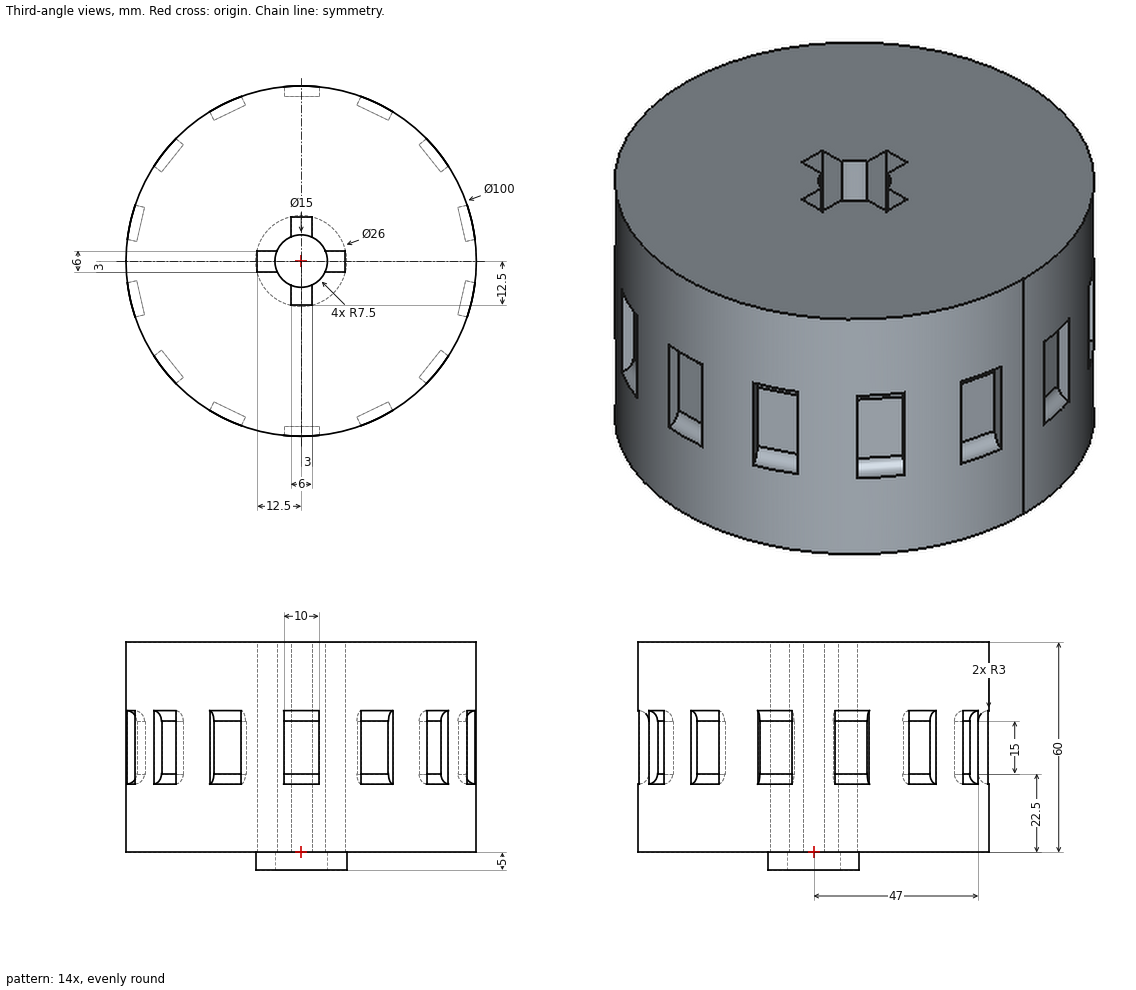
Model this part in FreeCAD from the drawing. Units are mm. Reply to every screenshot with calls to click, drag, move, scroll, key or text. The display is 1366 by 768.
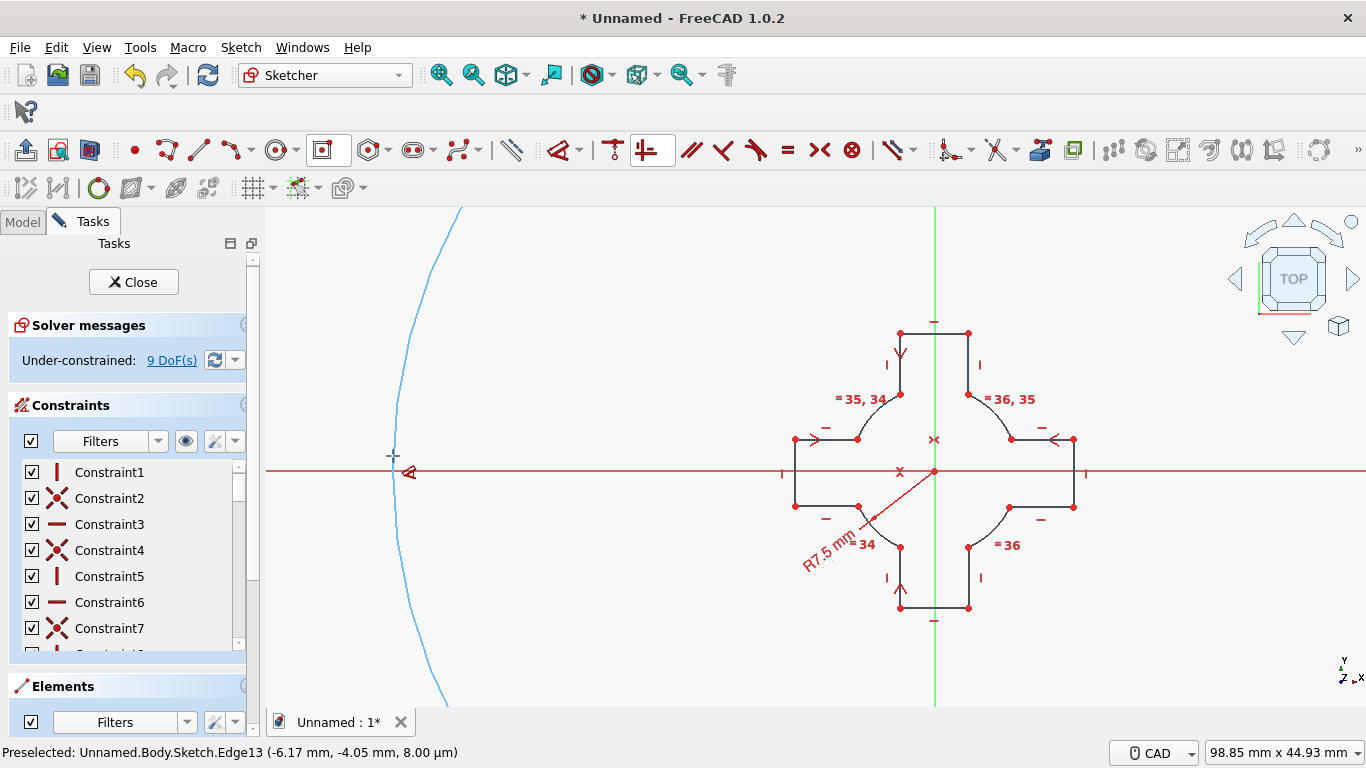
click(393, 456)
click(361, 455)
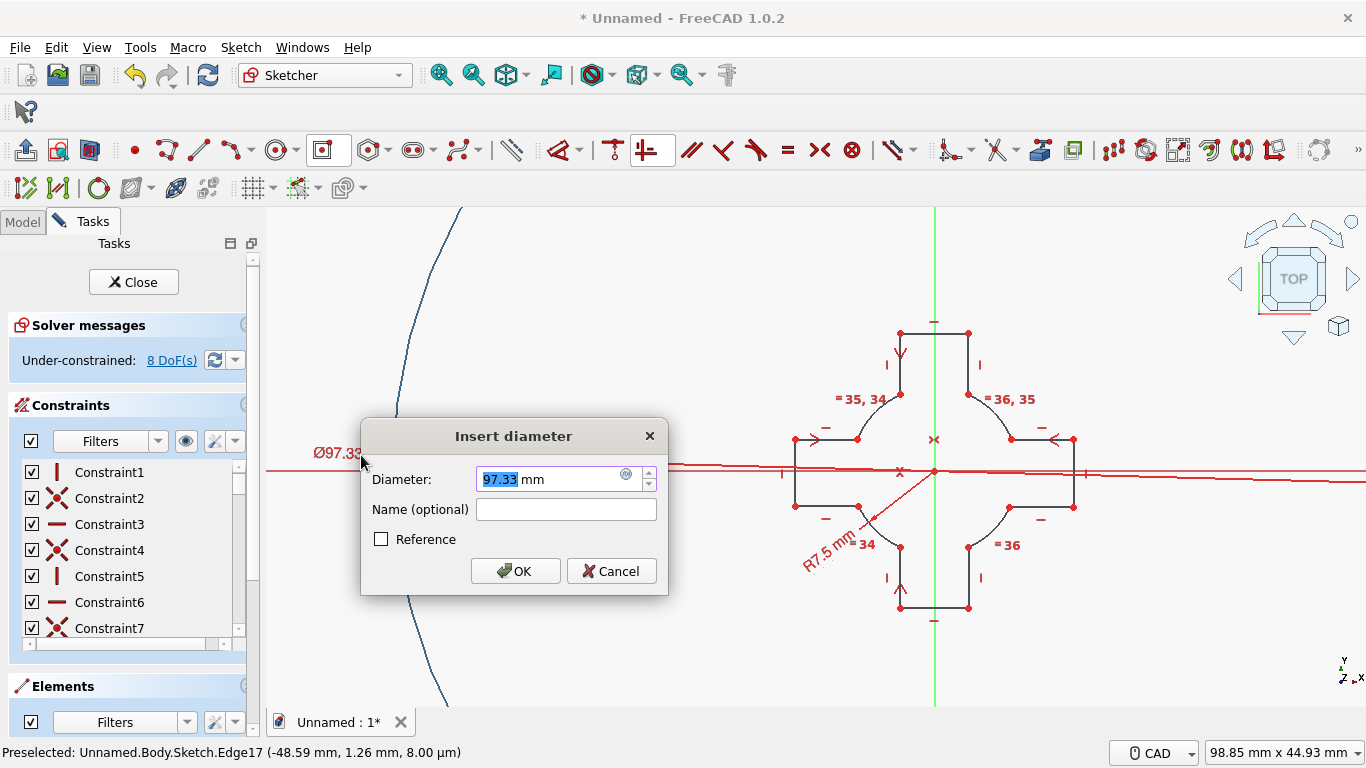
text(100)
key(Return)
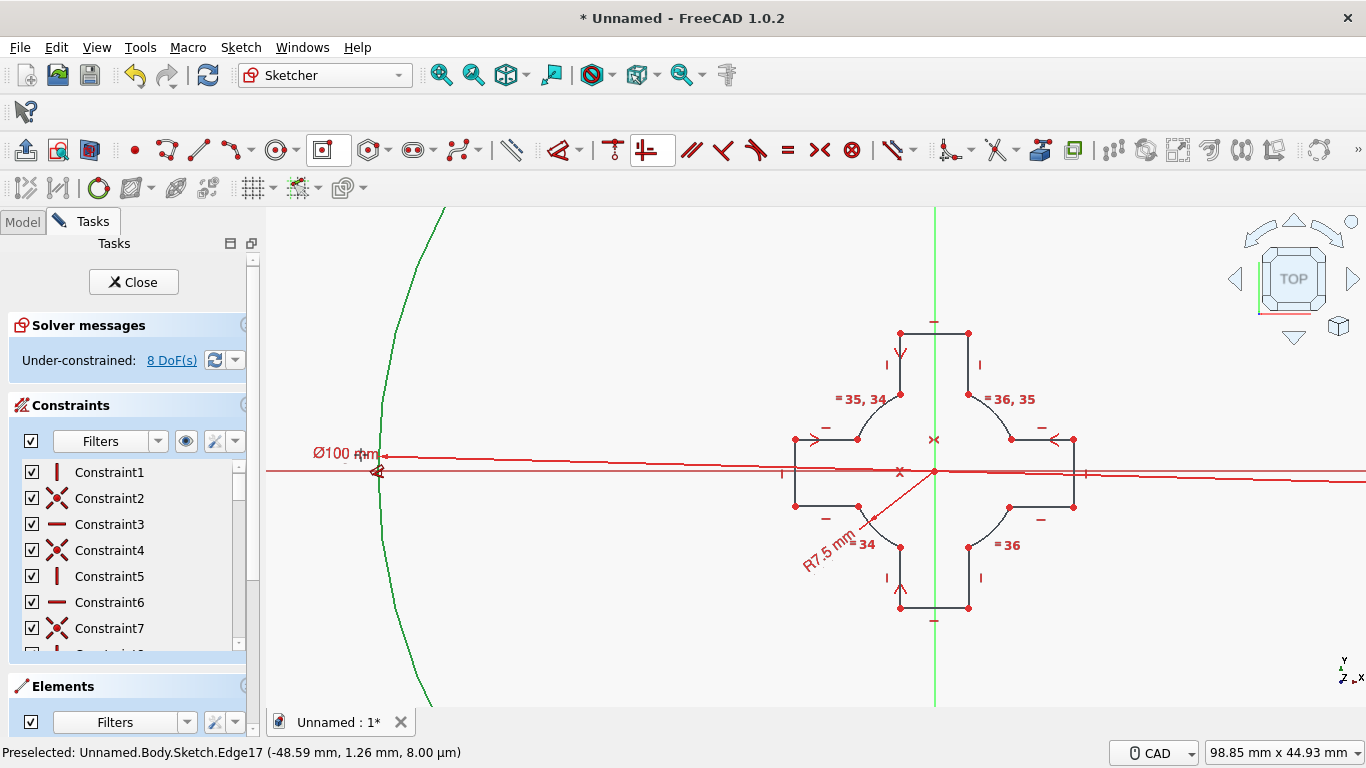
click(948, 608)
click(919, 642)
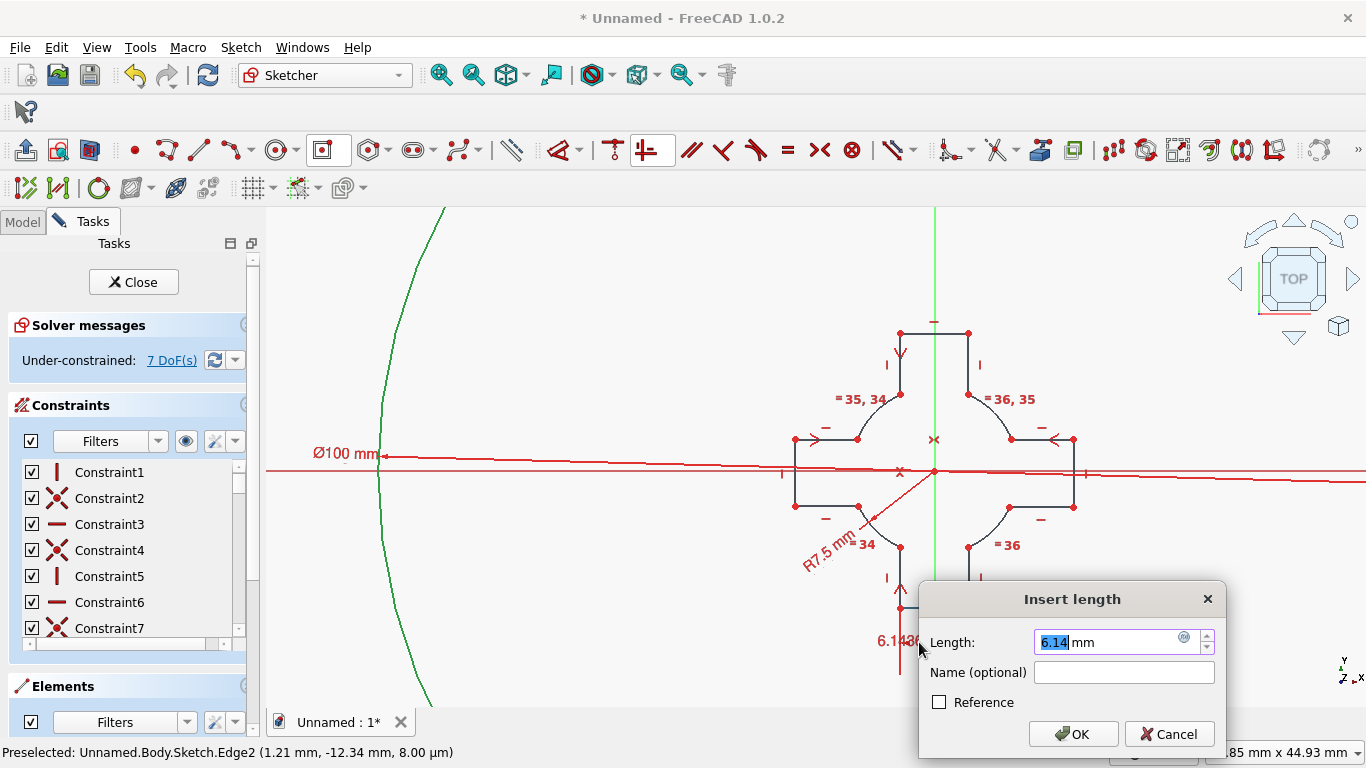
text(6)
key(Return)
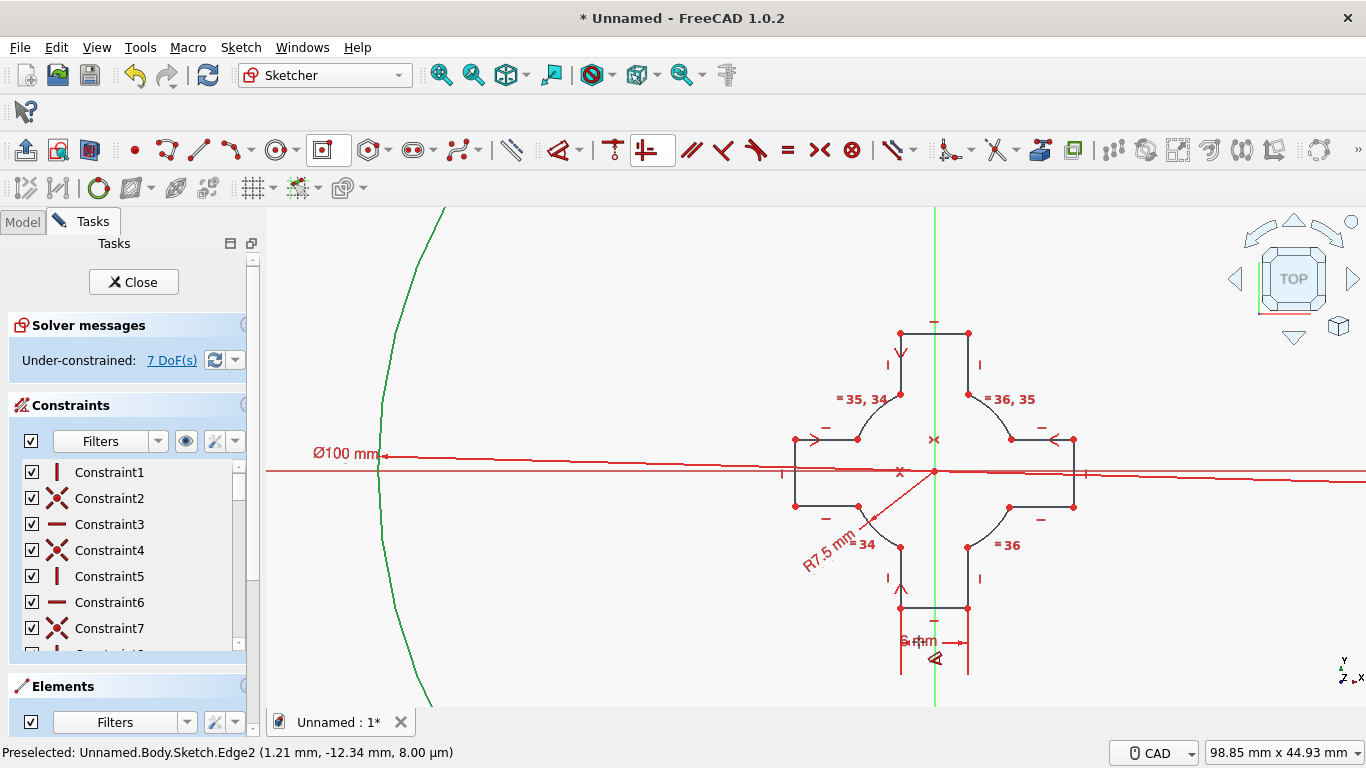
click(795, 486)
click(761, 458)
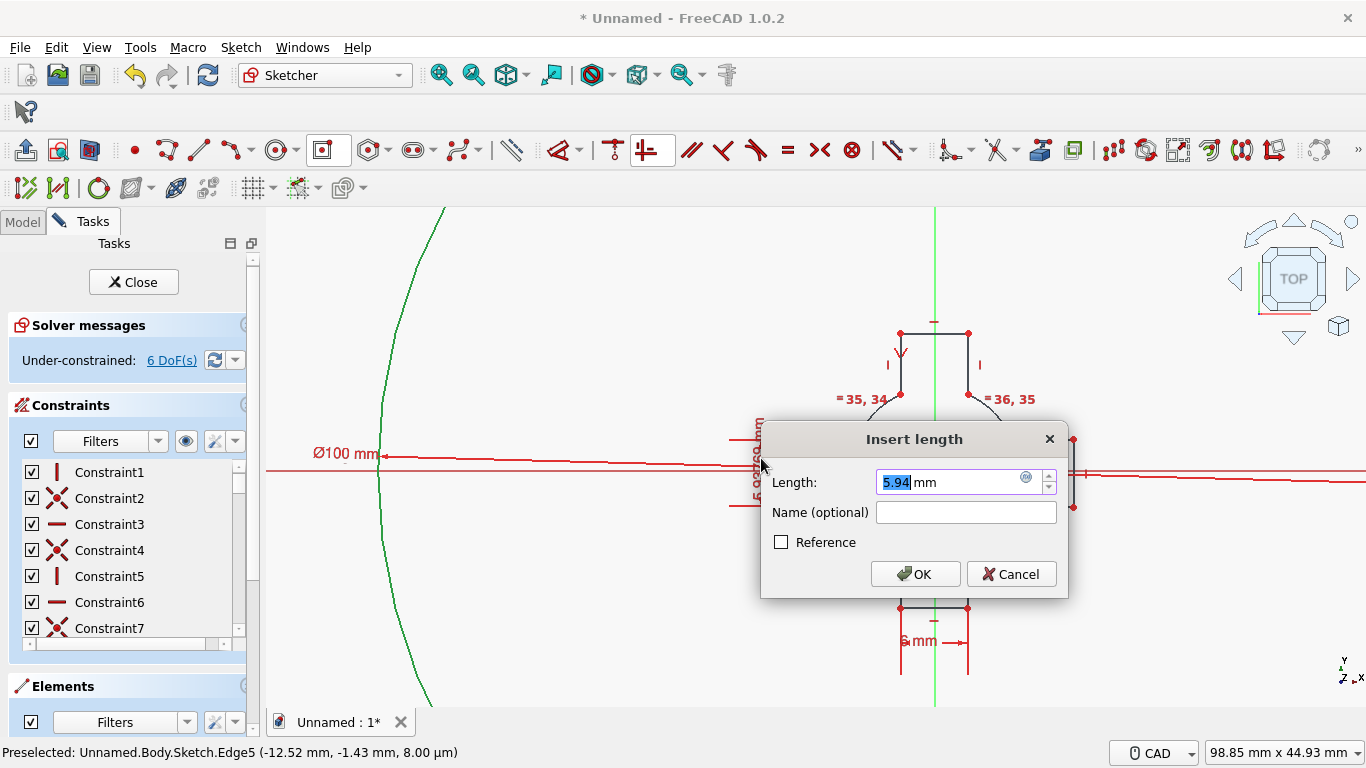
text(6)
key(Return)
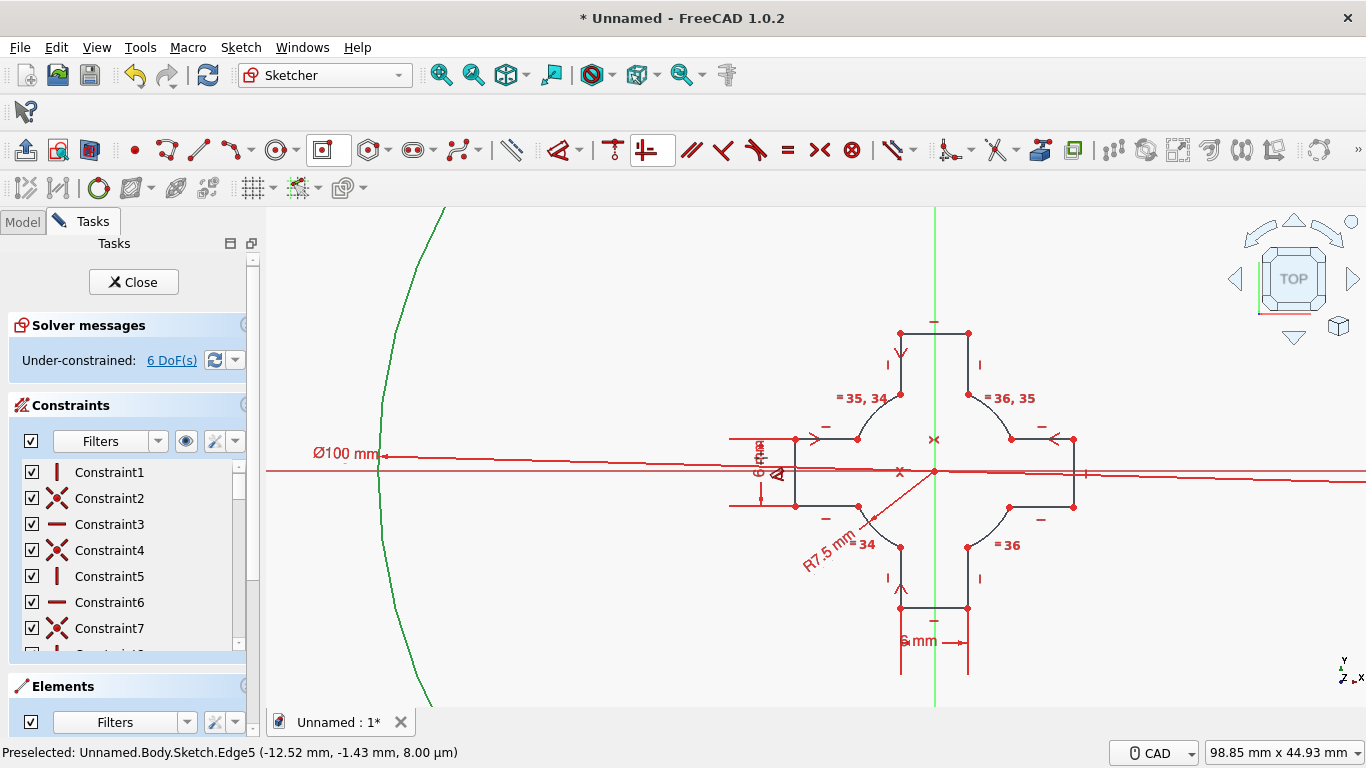
click(921, 334)
click(919, 300)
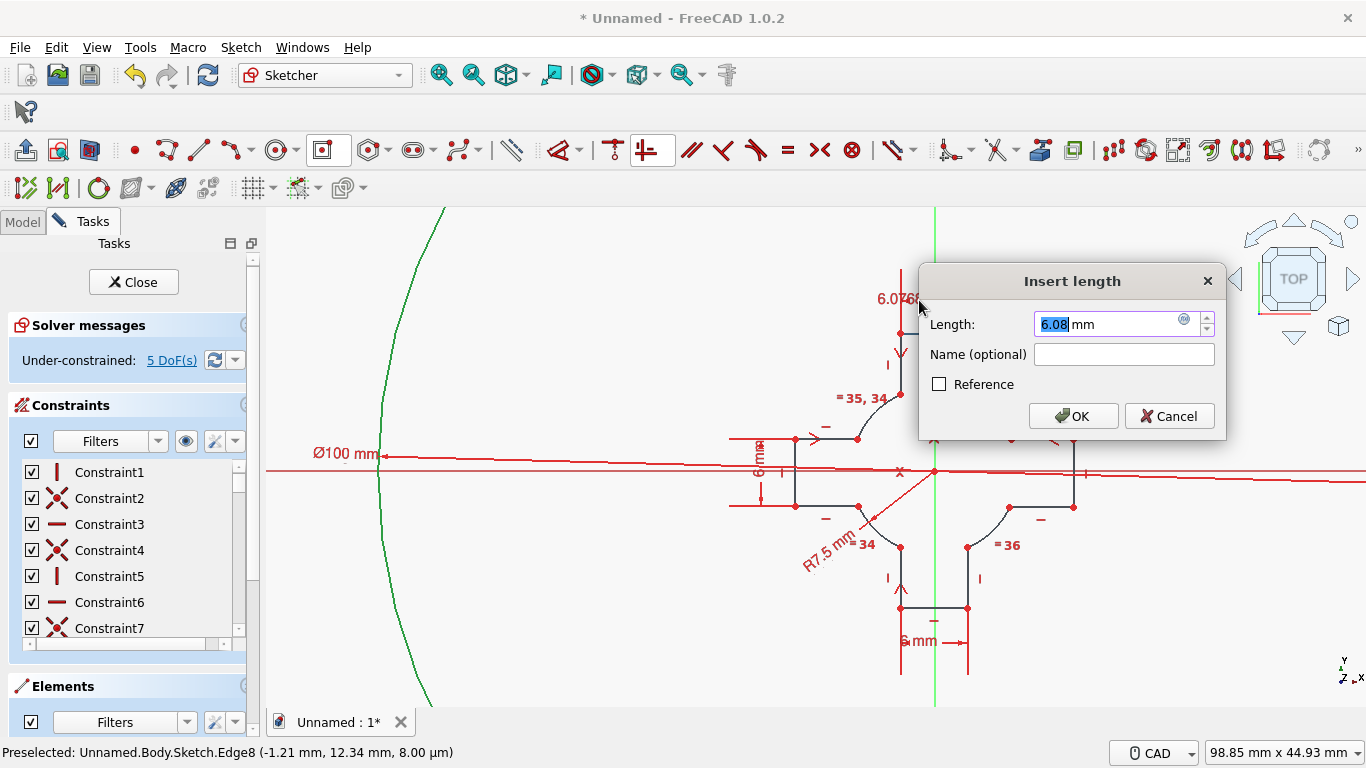
text(6)
key(Return)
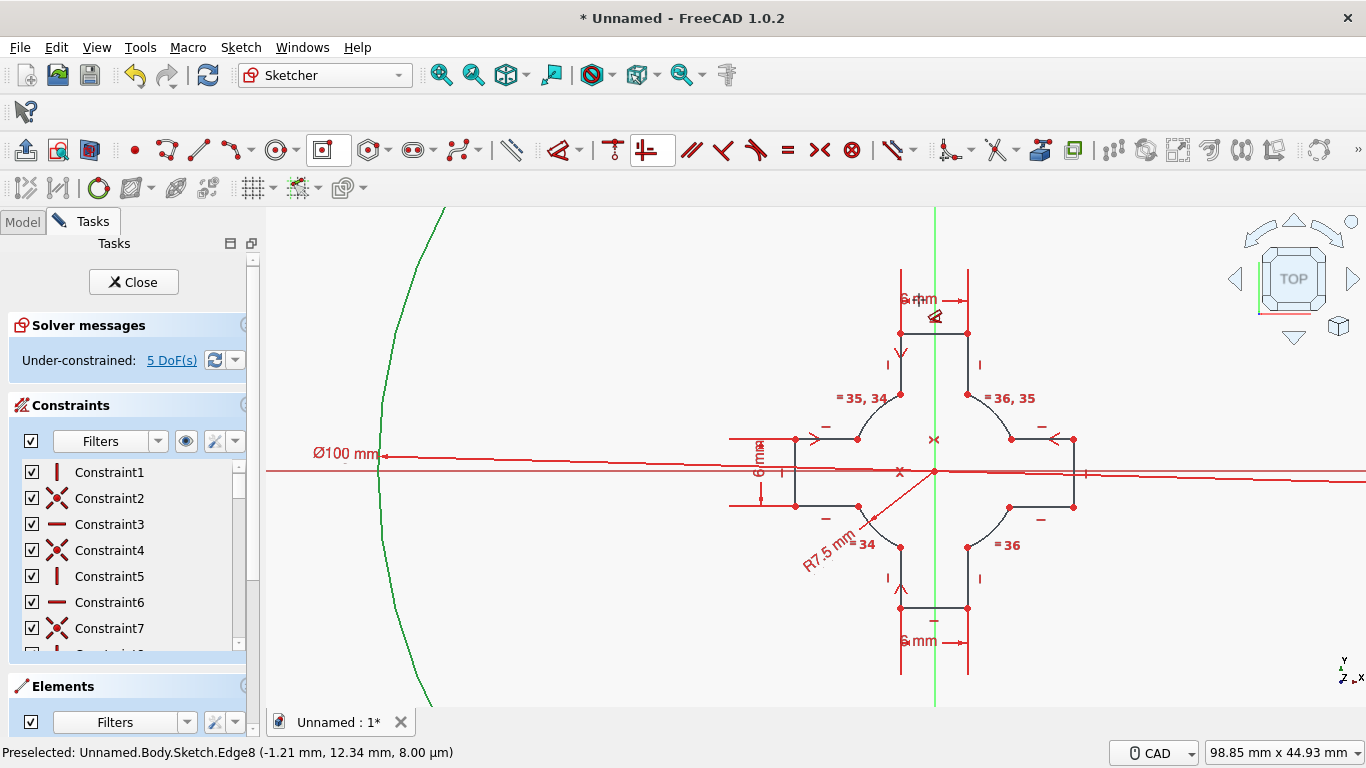
click(1074, 460)
click(1108, 458)